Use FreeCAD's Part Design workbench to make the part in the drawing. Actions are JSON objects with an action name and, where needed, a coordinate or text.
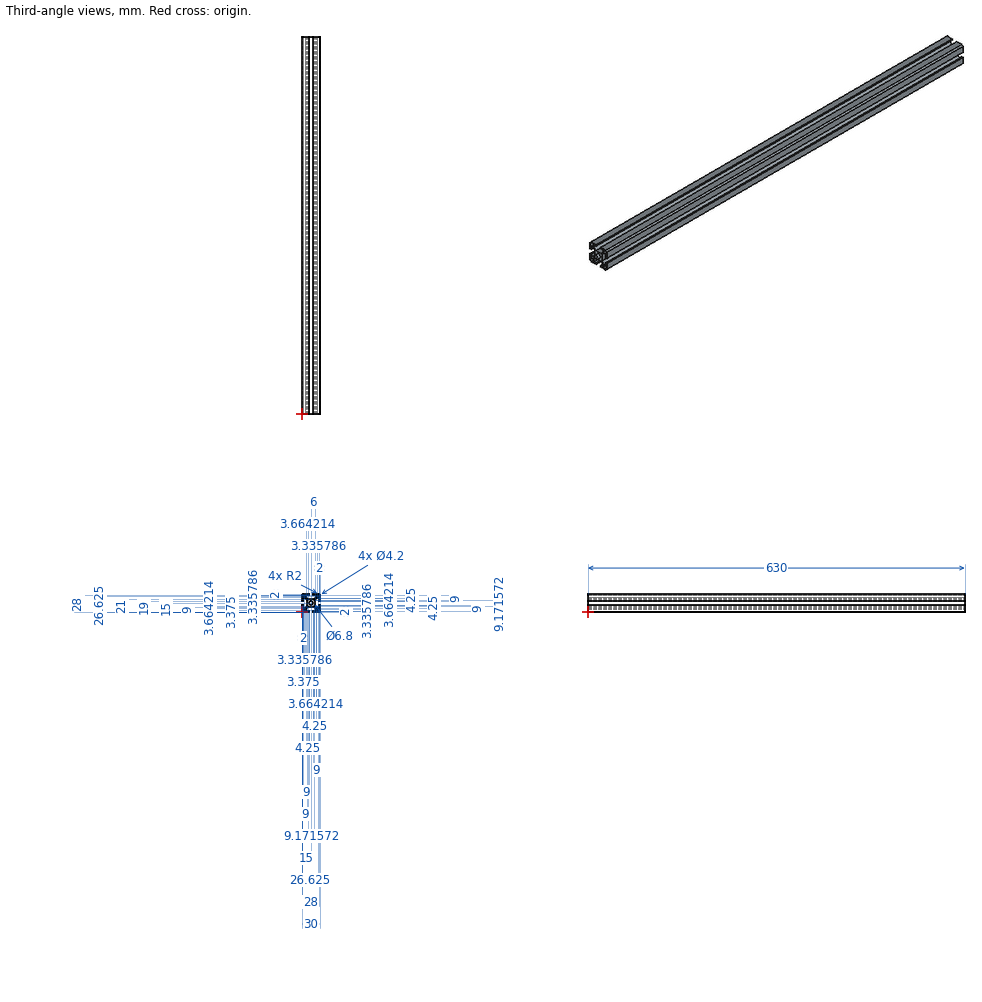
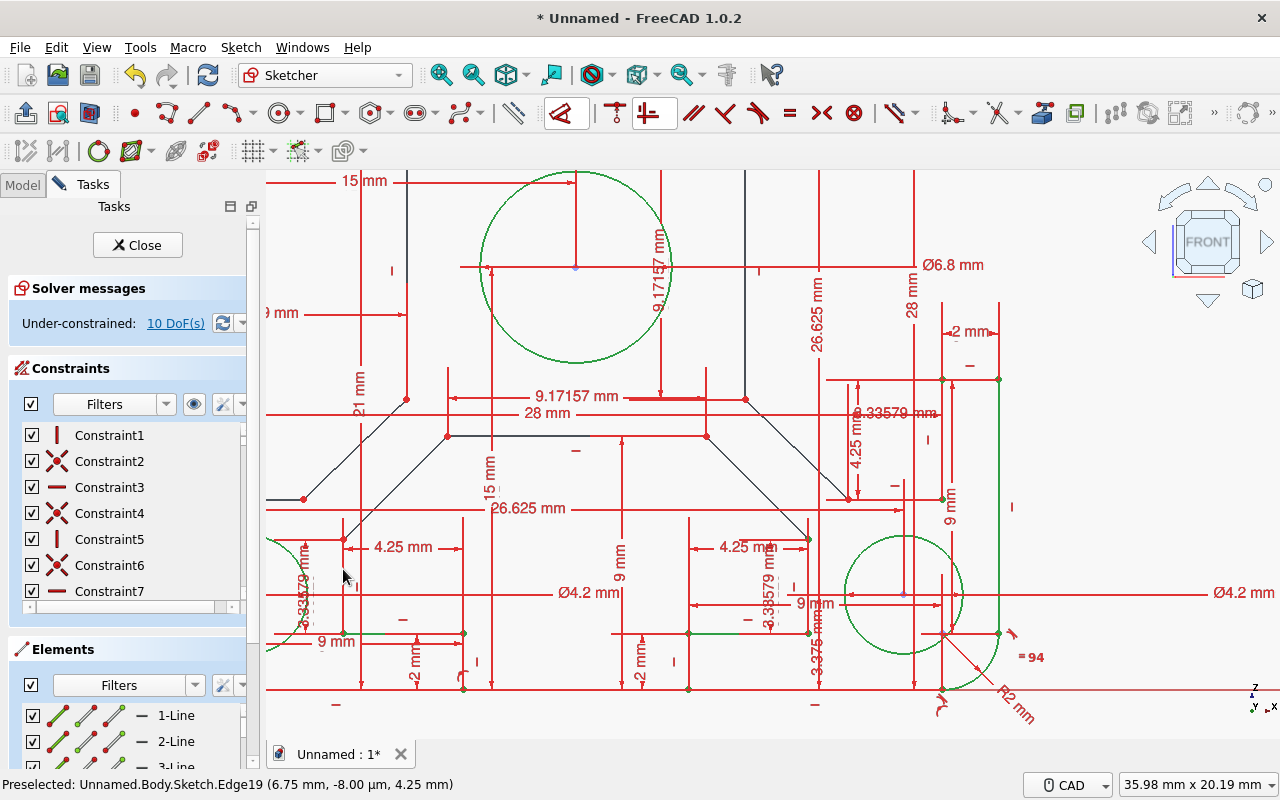
{"action": "scroll", "coordinate": [809, 607], "scroll_direction": "down", "scroll_amount": 4}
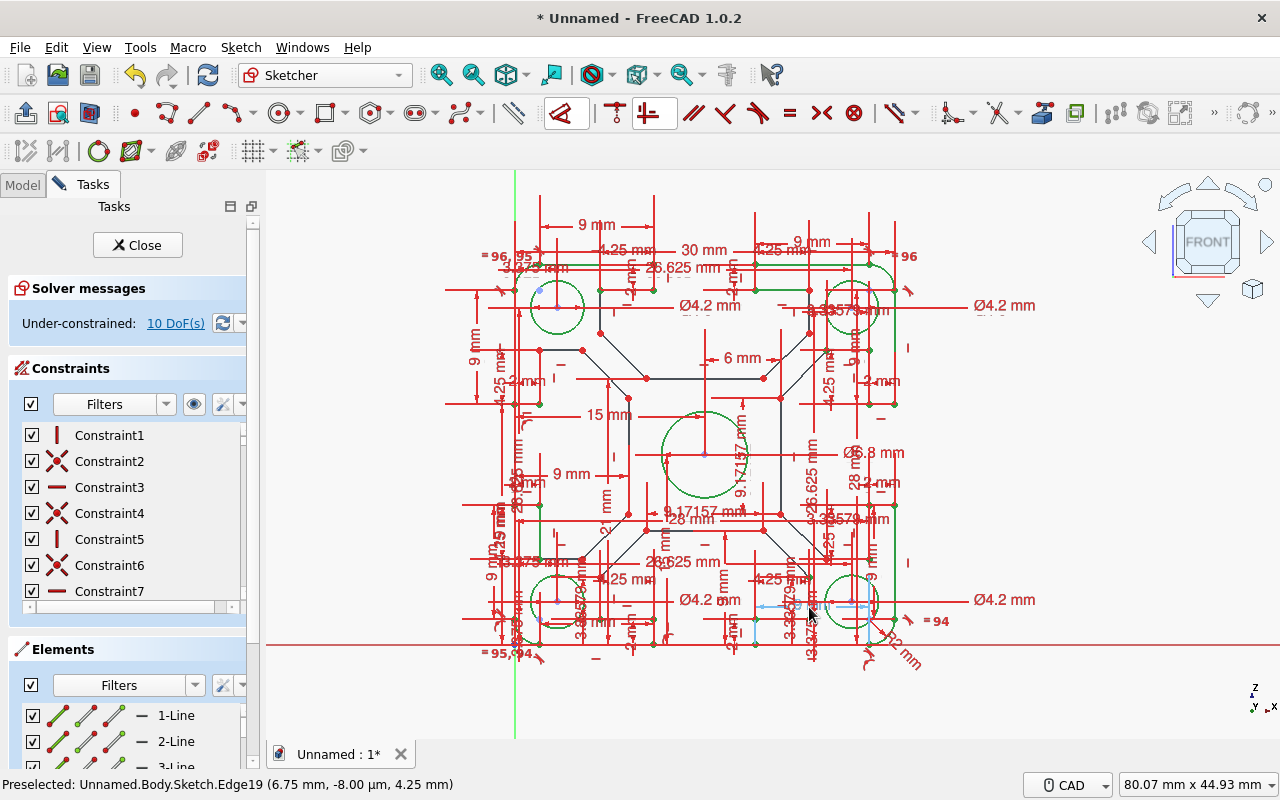
{"action": "left_click", "coordinate": [574, 559]}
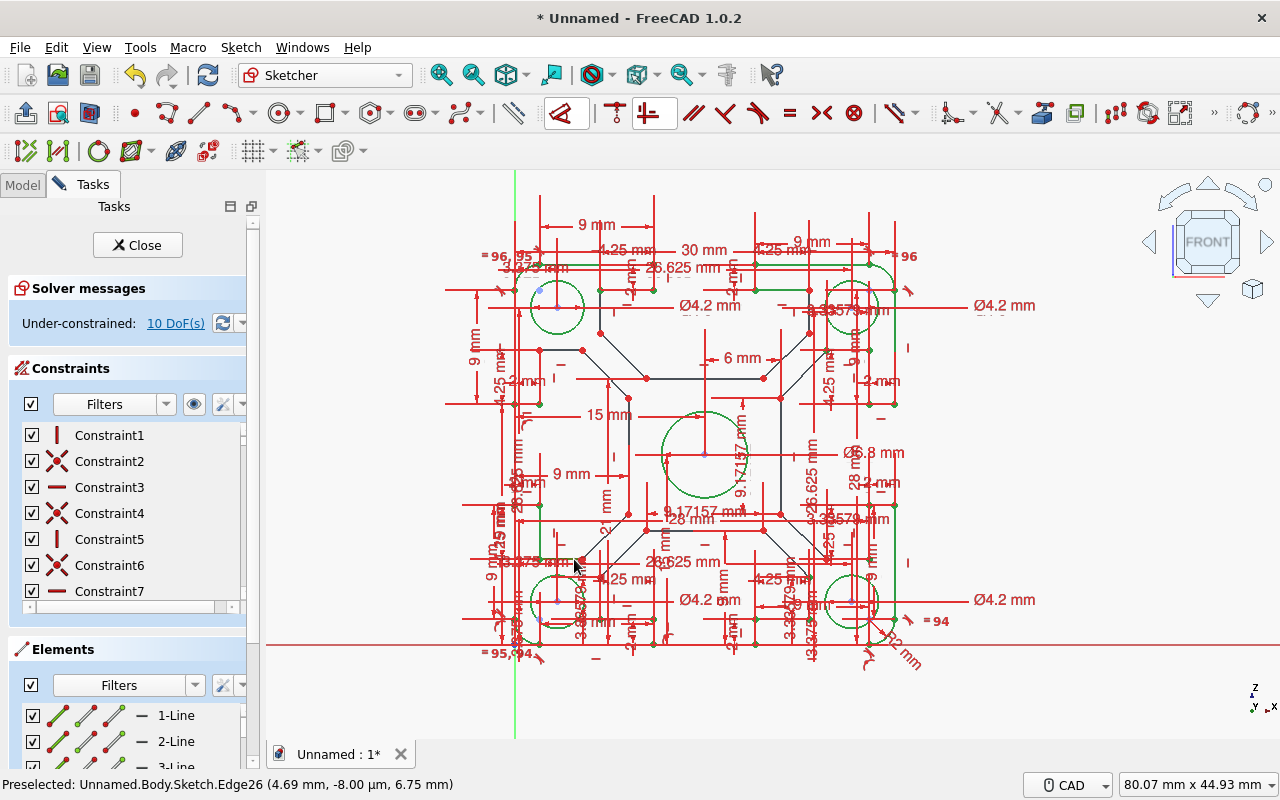
{"action": "left_click", "coordinate": [584, 114]}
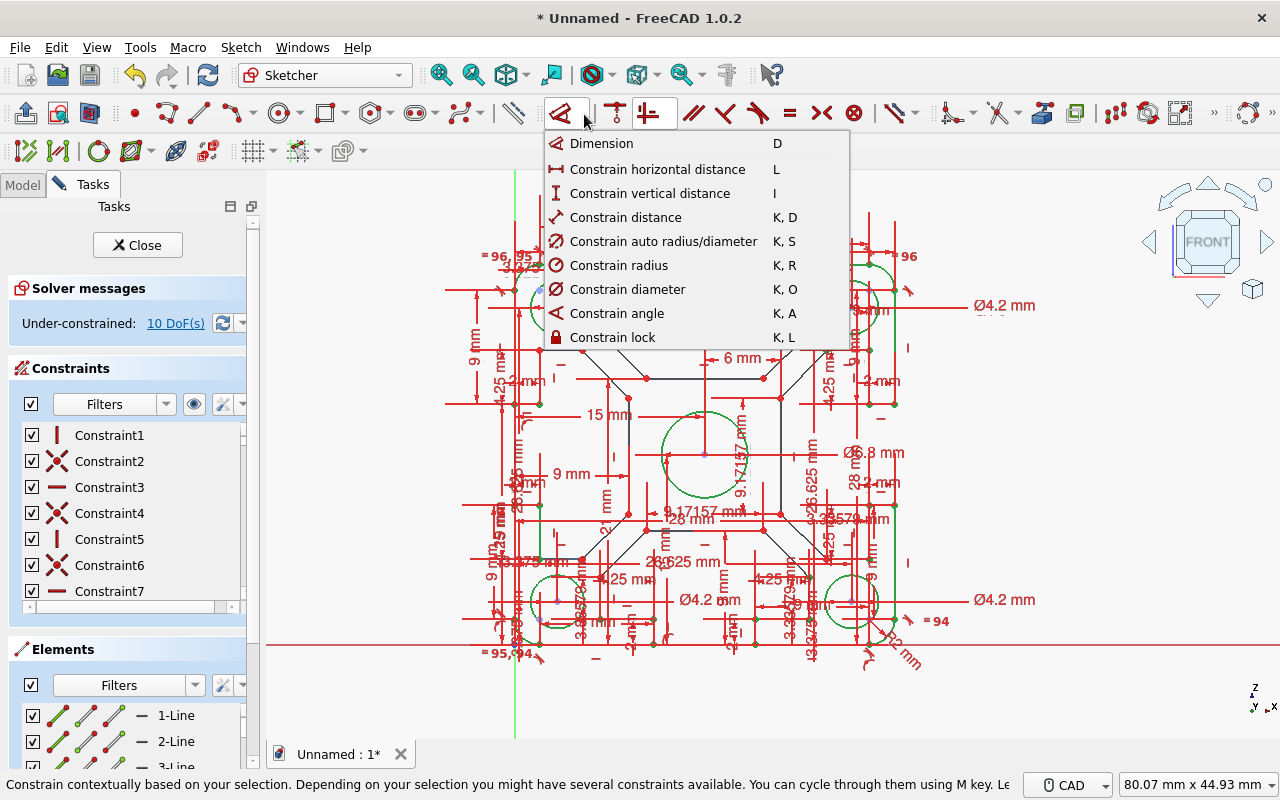
{"action": "left_click", "coordinate": [697, 169]}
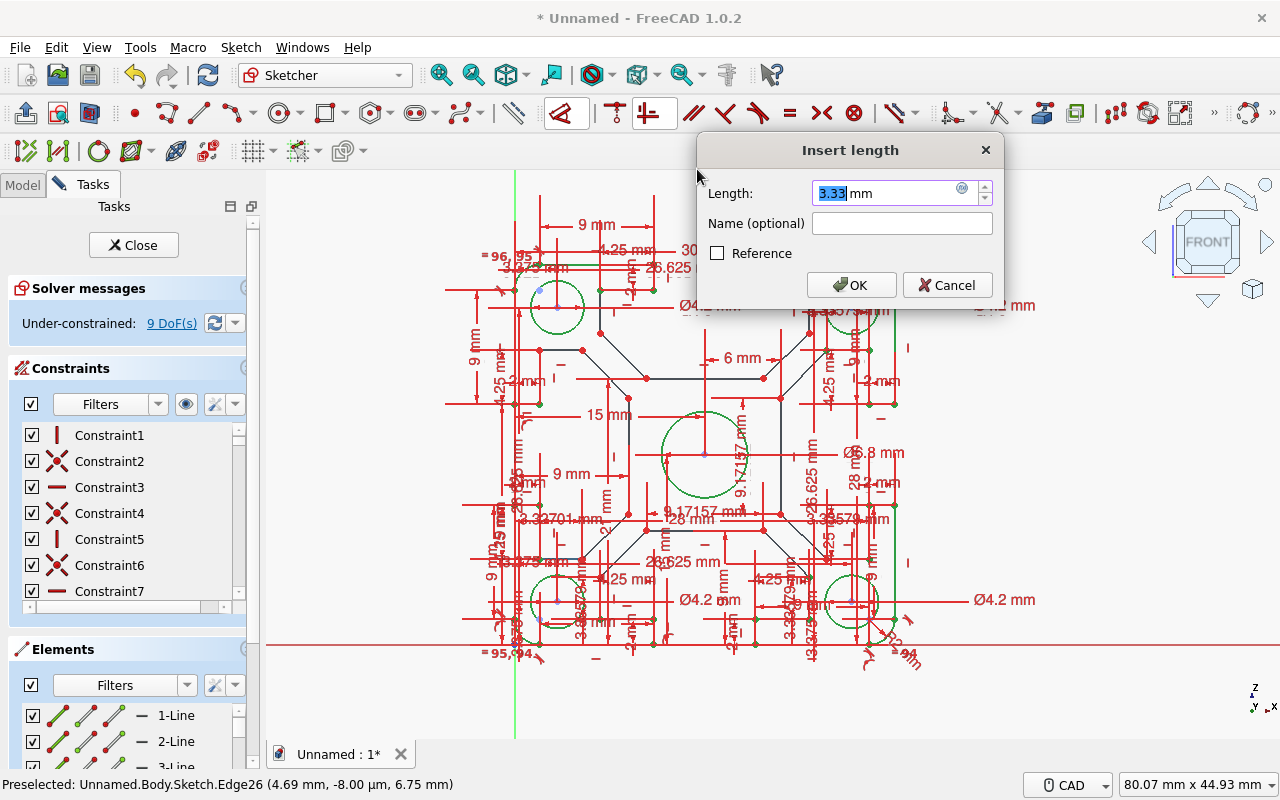
{"action": "type", "text": "3.335786"}
{"action": "key", "text": "Return"}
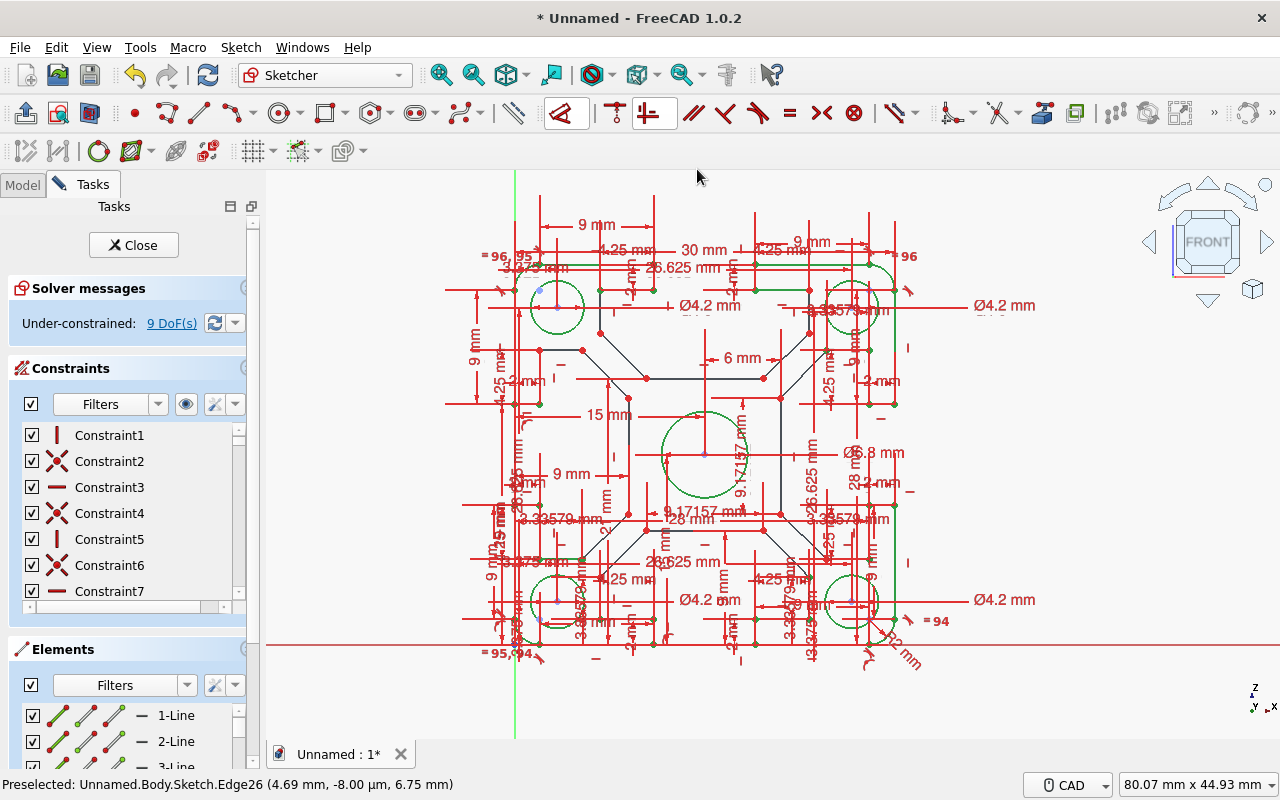
{"action": "left_click", "coordinate": [629, 479]}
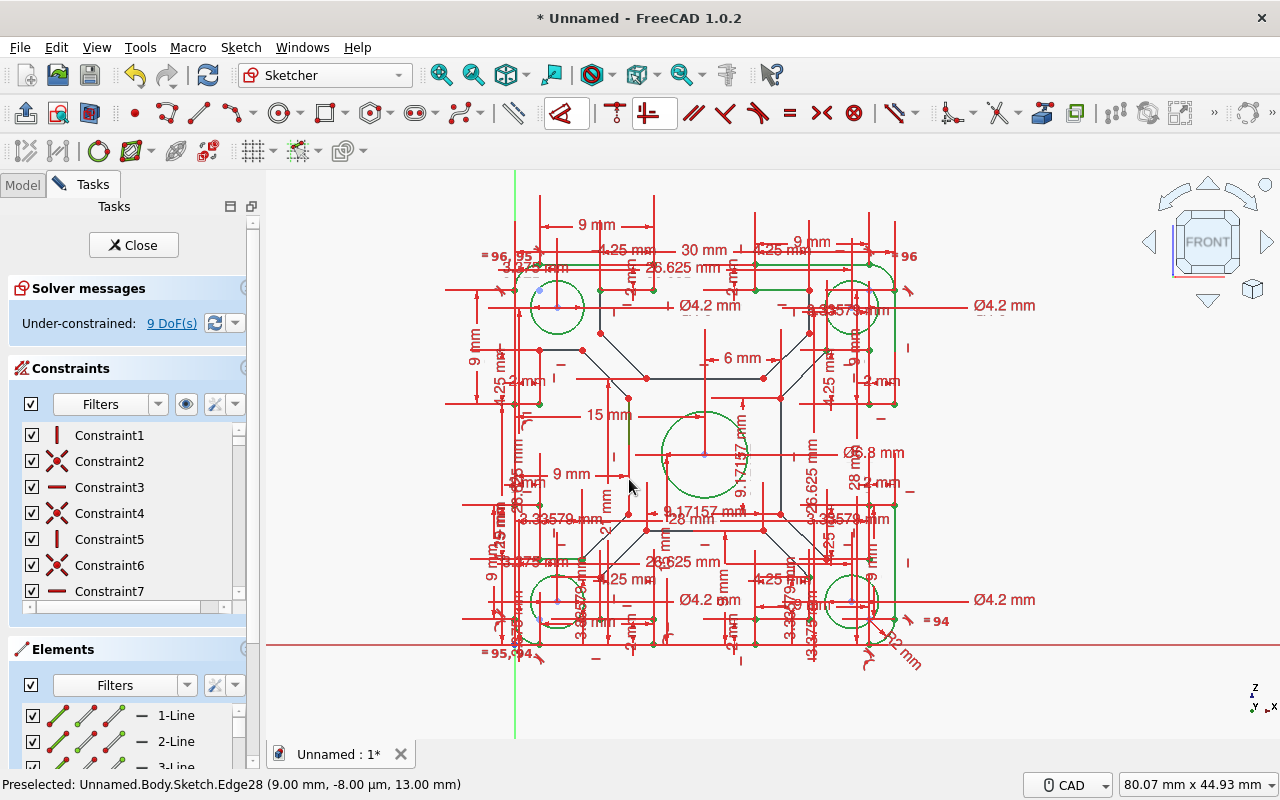
{"action": "key", "text": "i"}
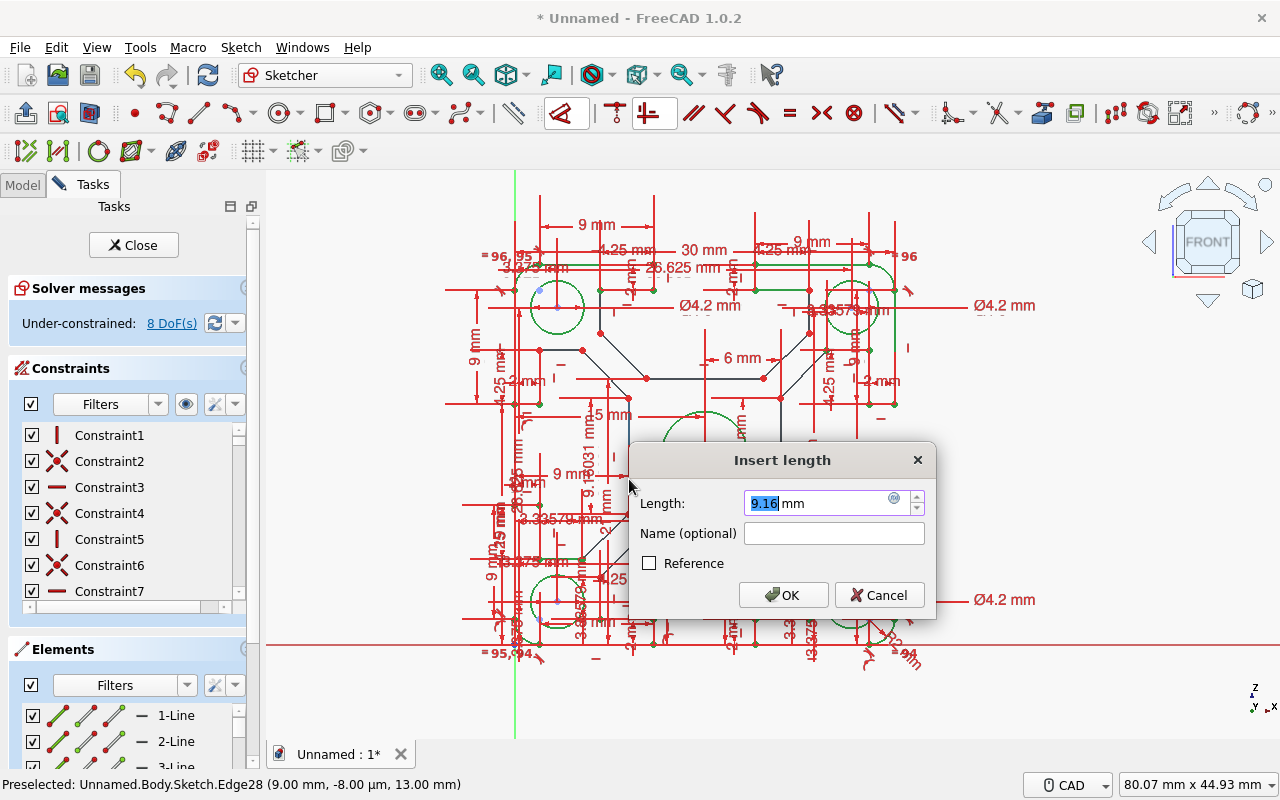
{"action": "type", "text": "9.171572"}
{"action": "key", "text": "Return"}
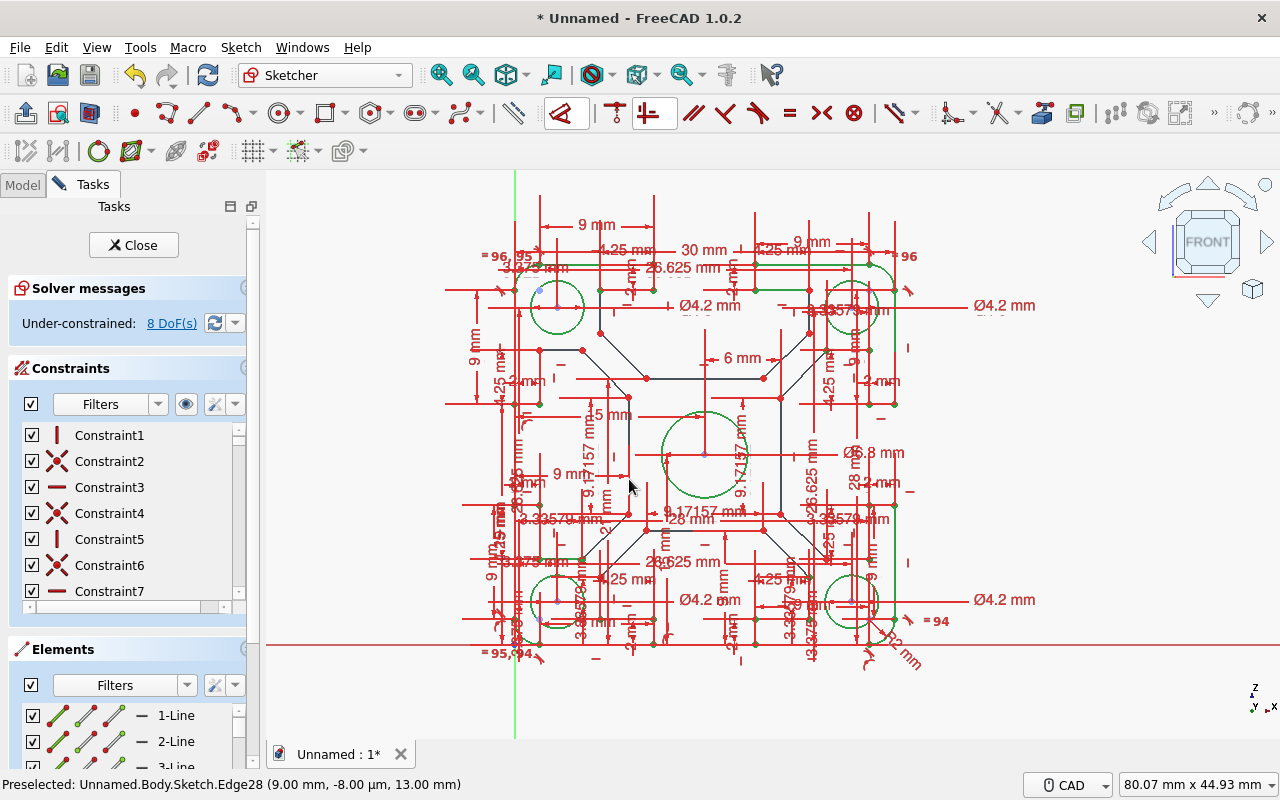
{"action": "left_click", "coordinate": [569, 350]}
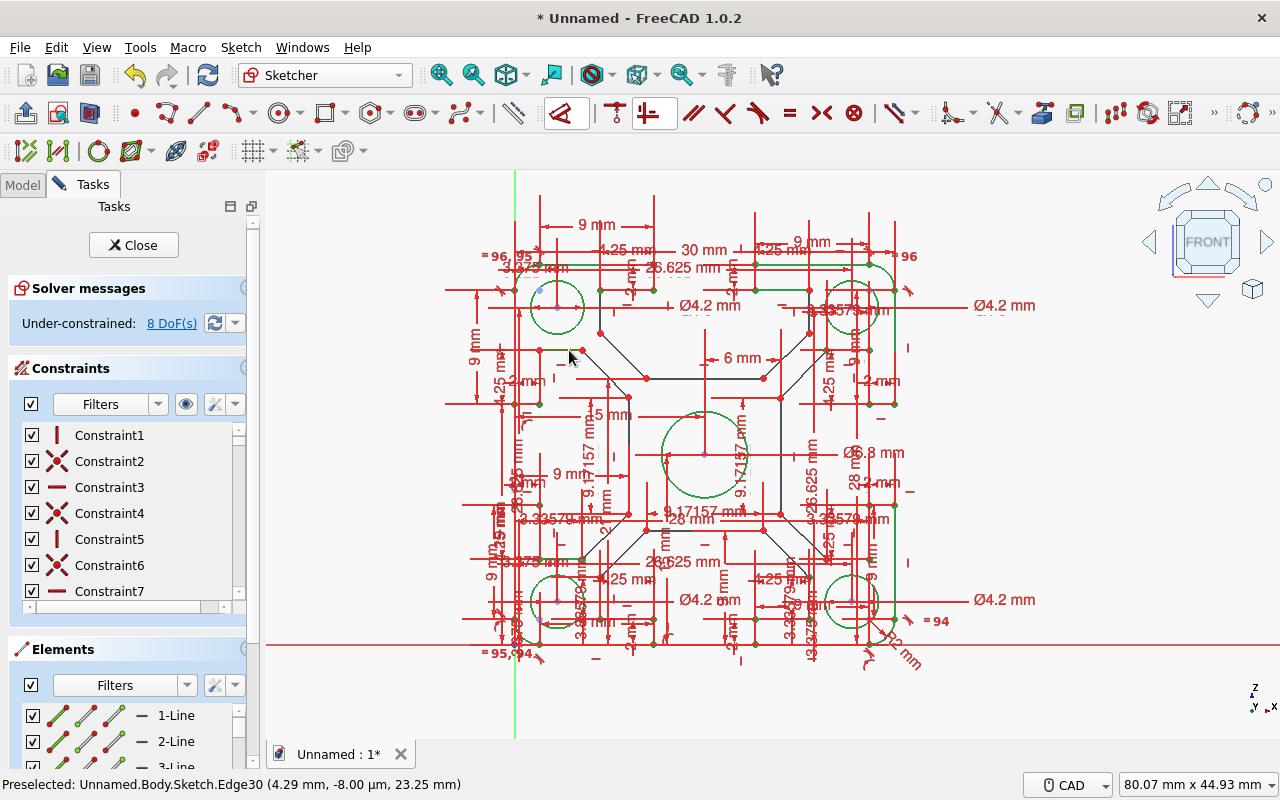
{"action": "left_click", "coordinate": [584, 114]}